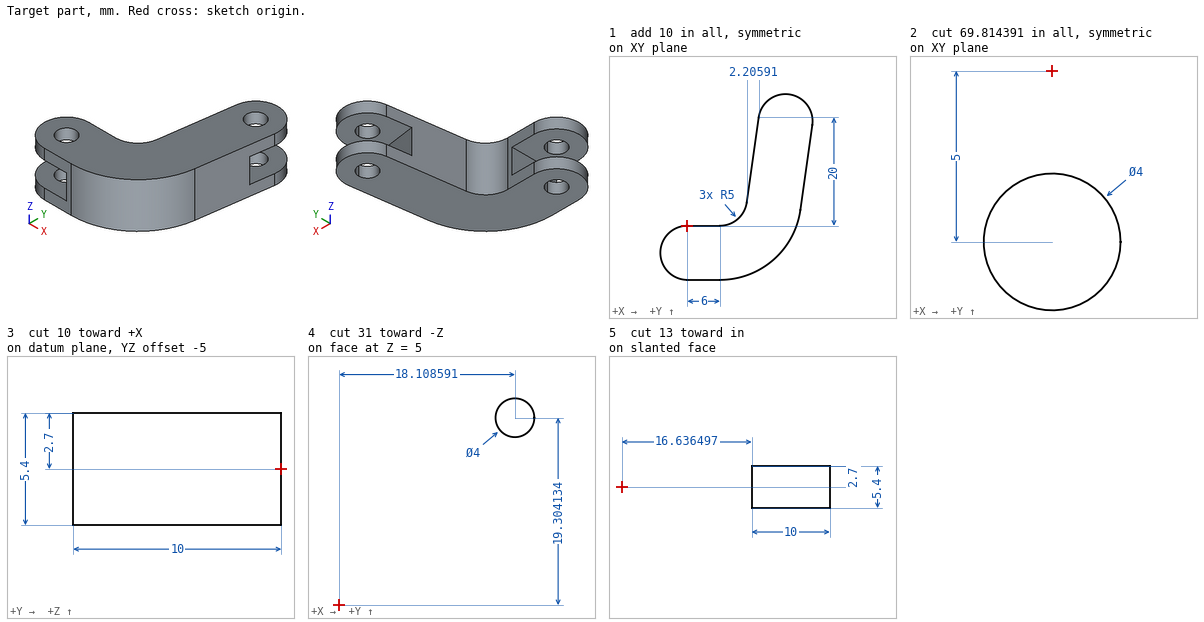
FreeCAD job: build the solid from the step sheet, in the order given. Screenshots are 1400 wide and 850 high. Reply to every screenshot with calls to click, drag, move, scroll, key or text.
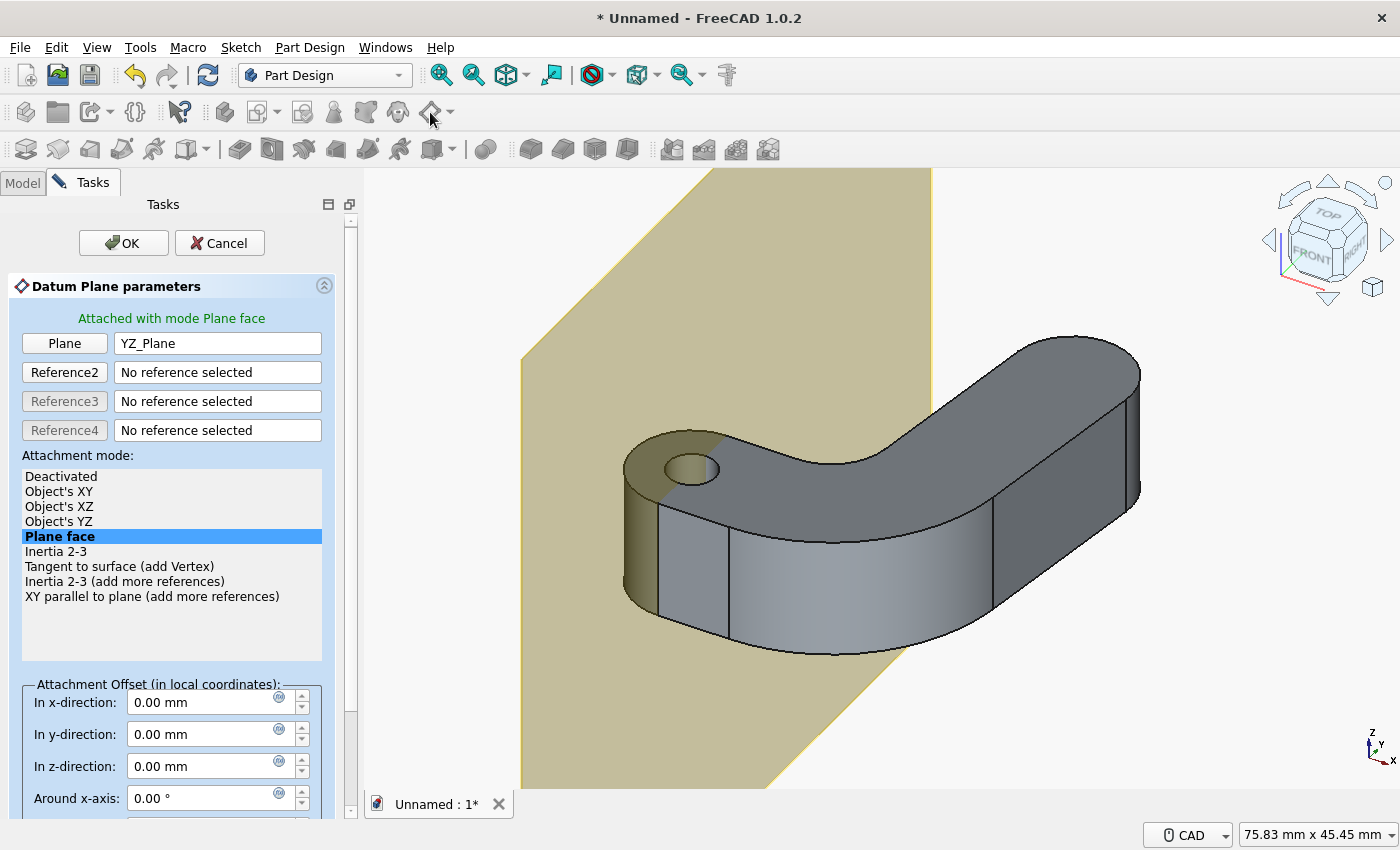
triple_click(210, 766)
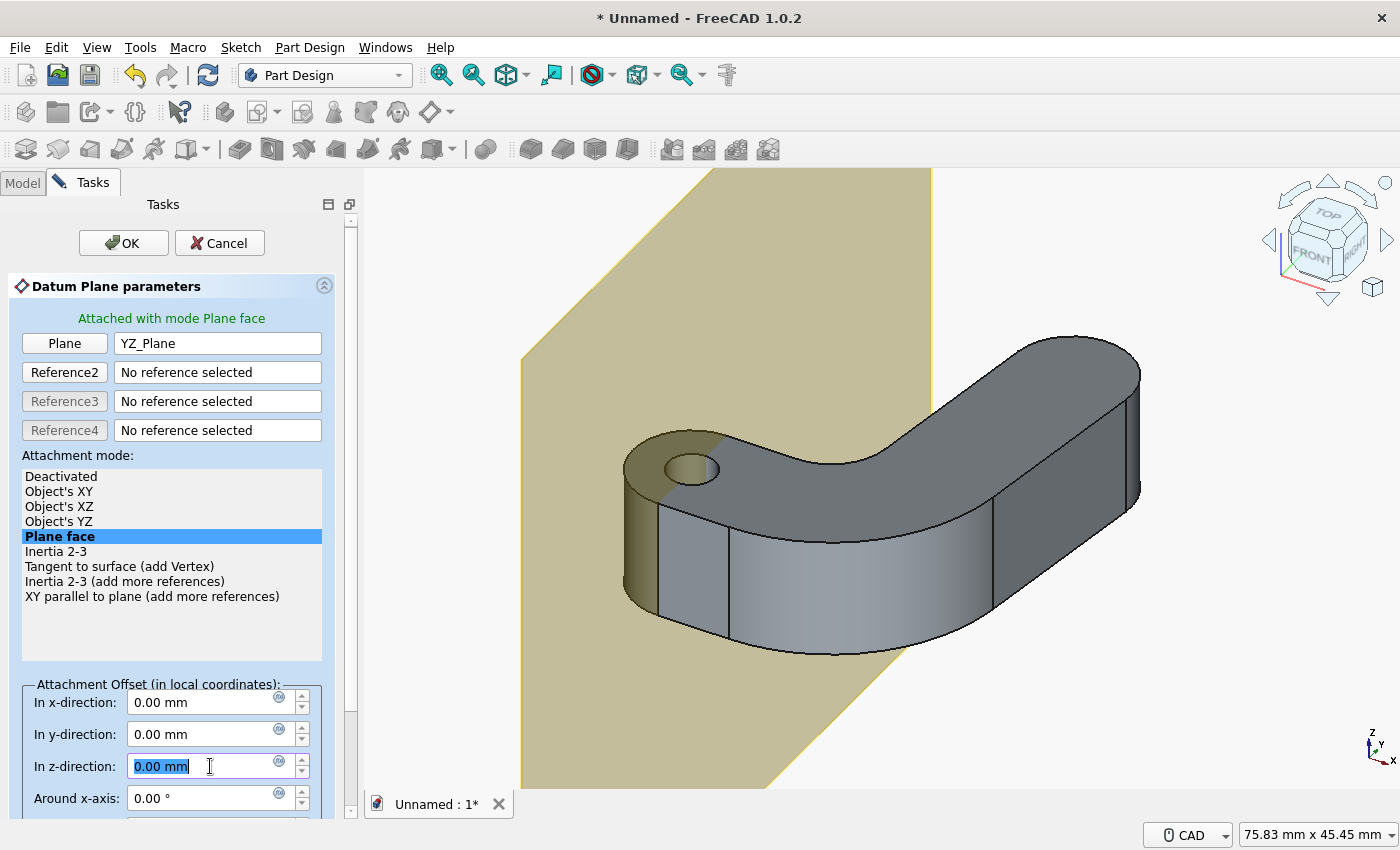
text(-5)
key(Tab)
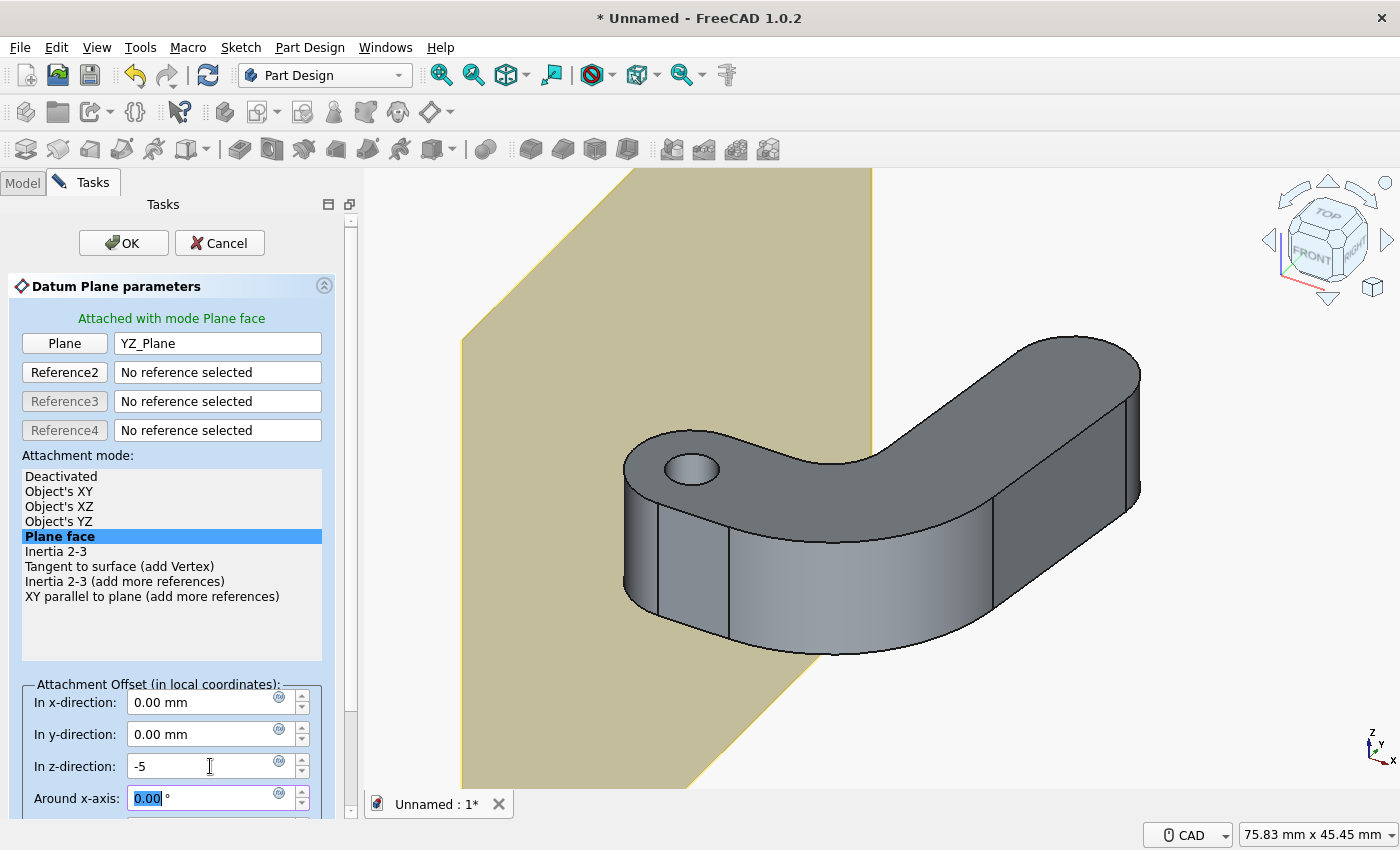
click(124, 243)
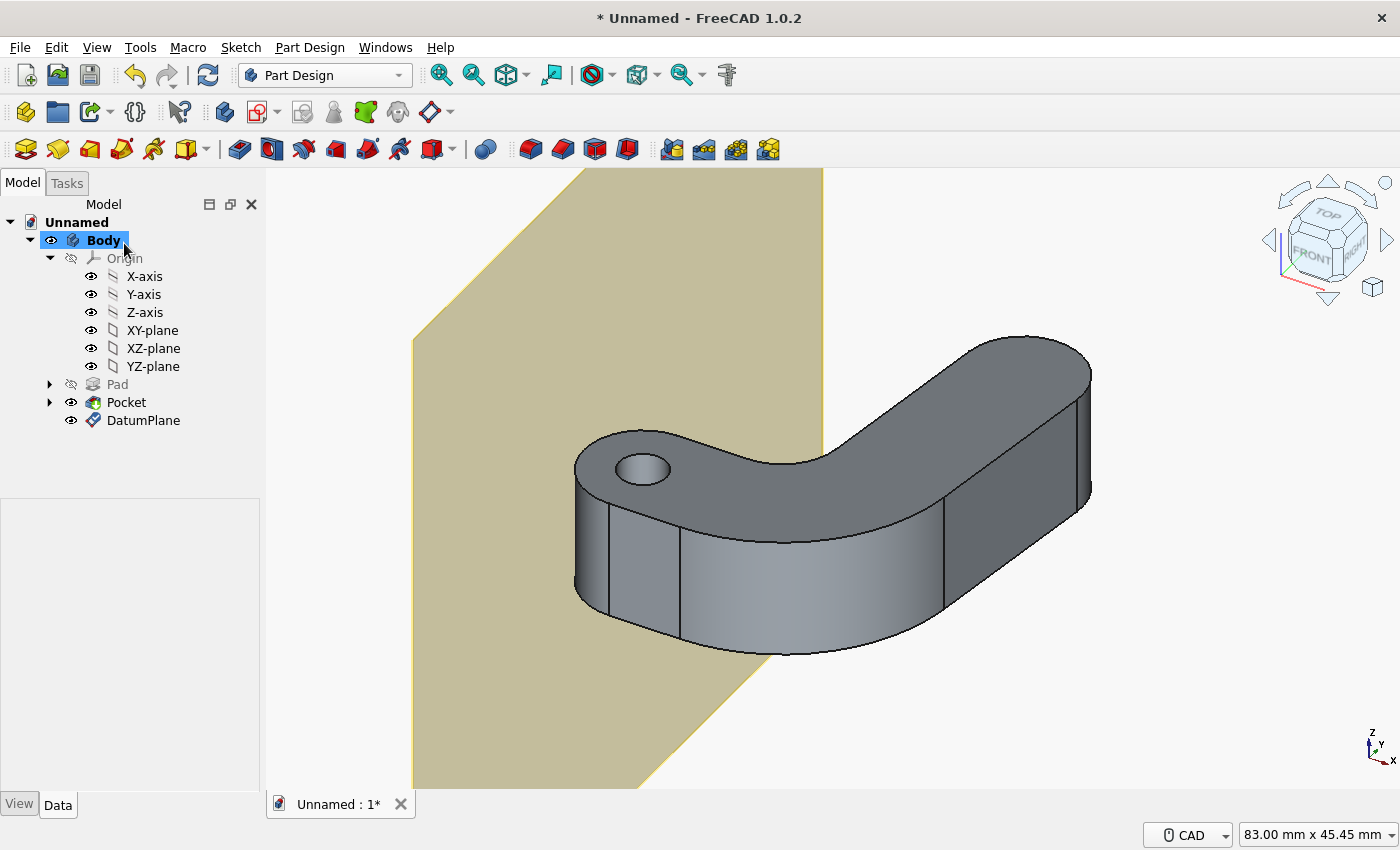
click(116, 420)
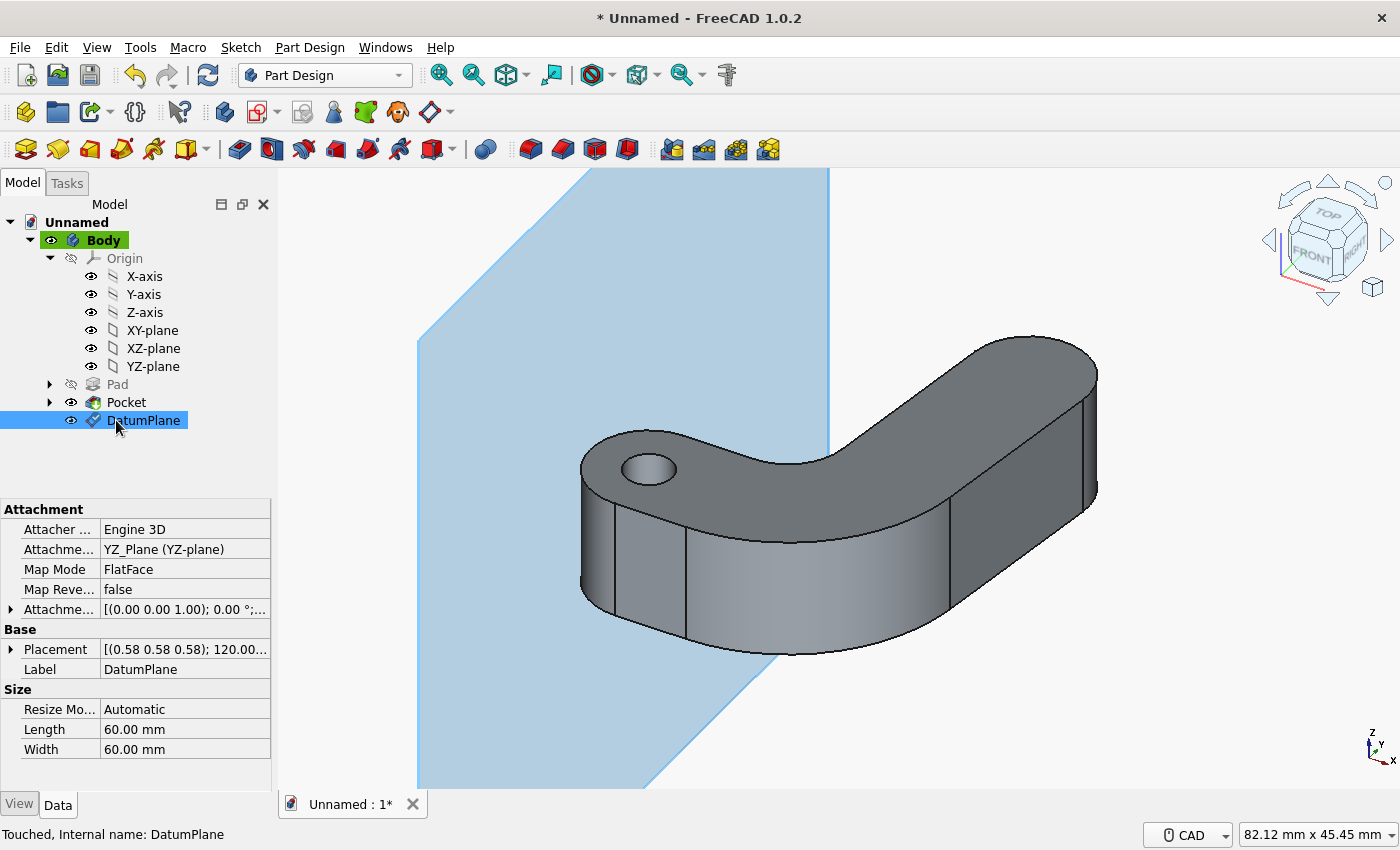
click(258, 112)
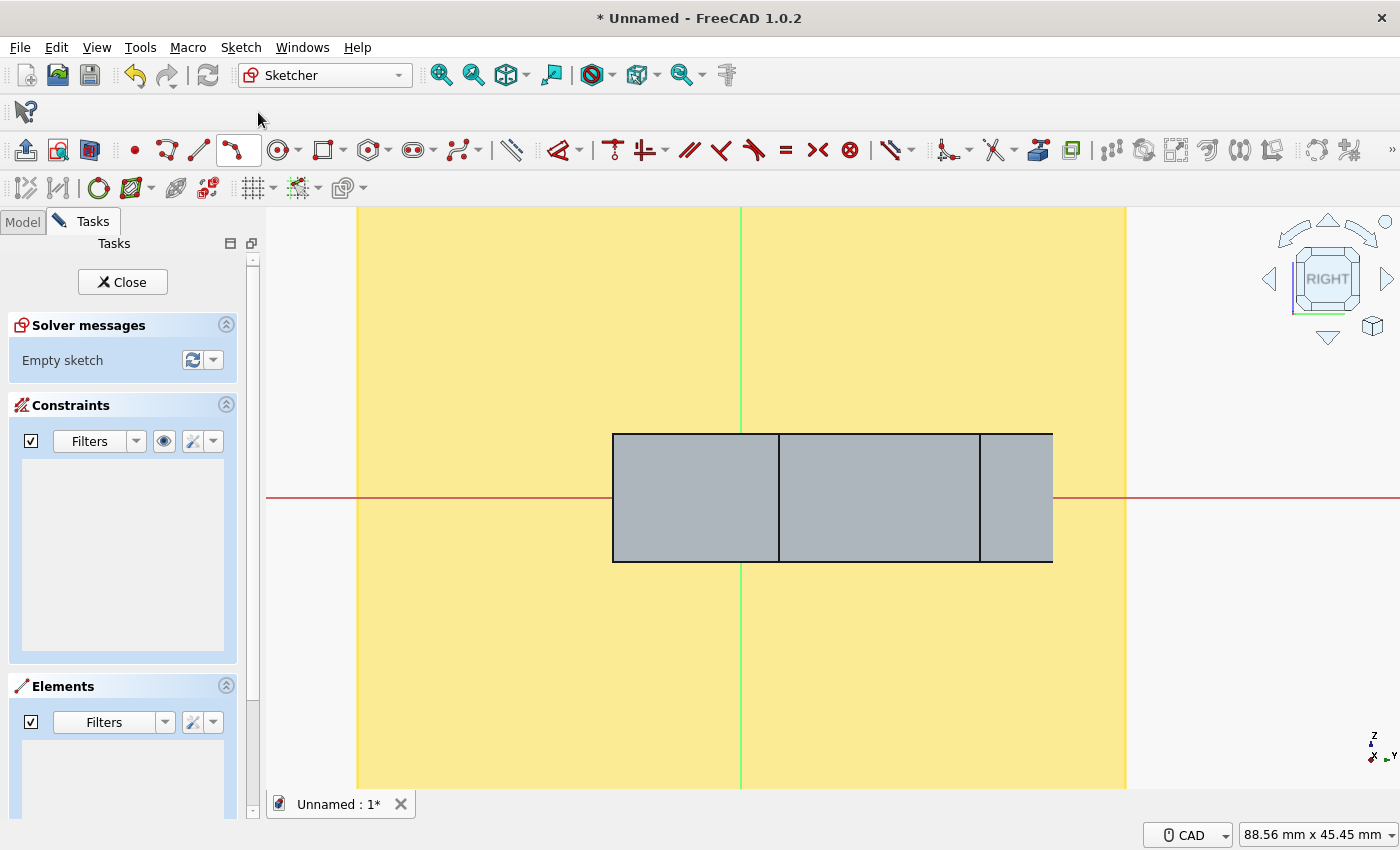
click(90, 150)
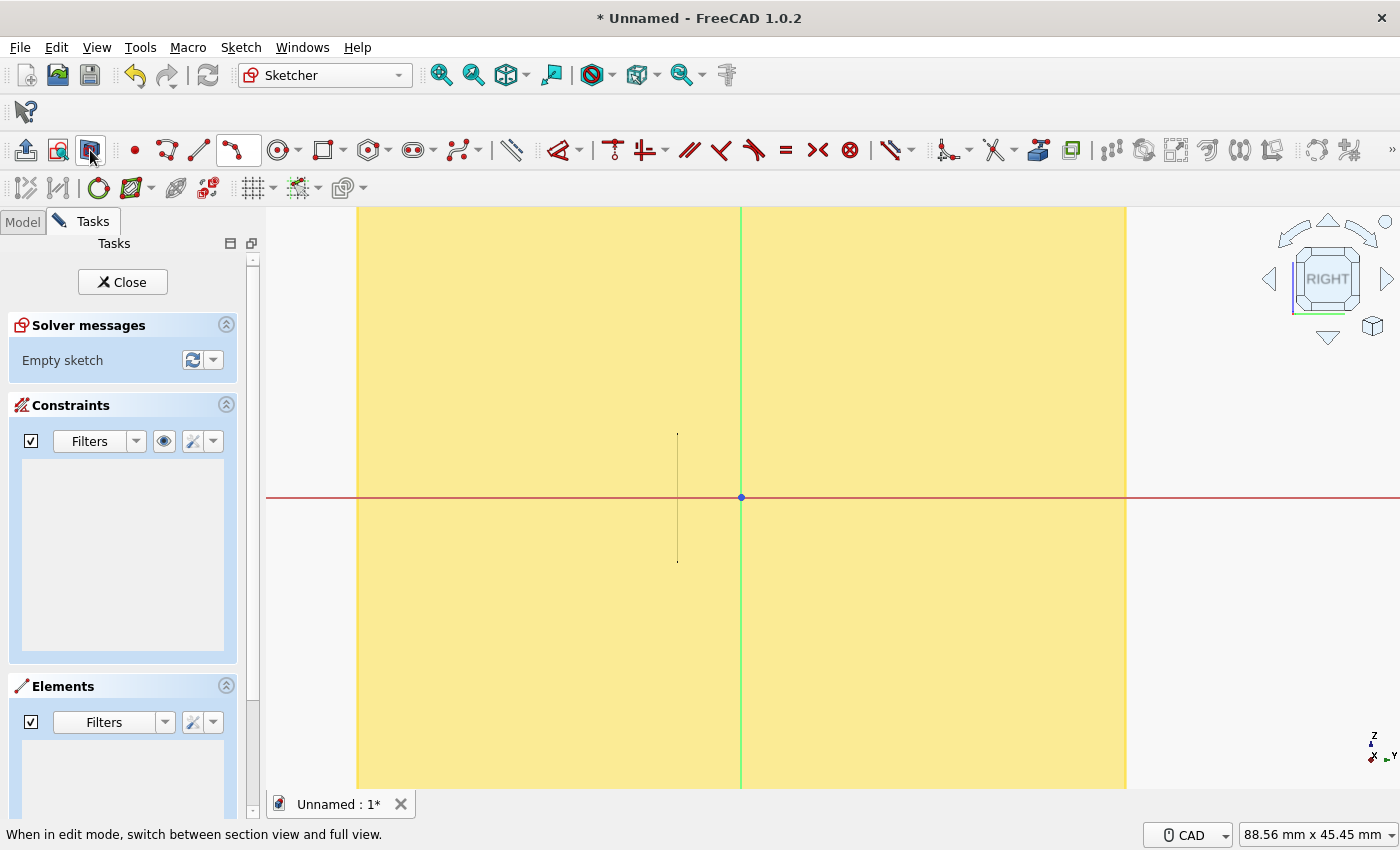
scroll(655, 498, up, 8)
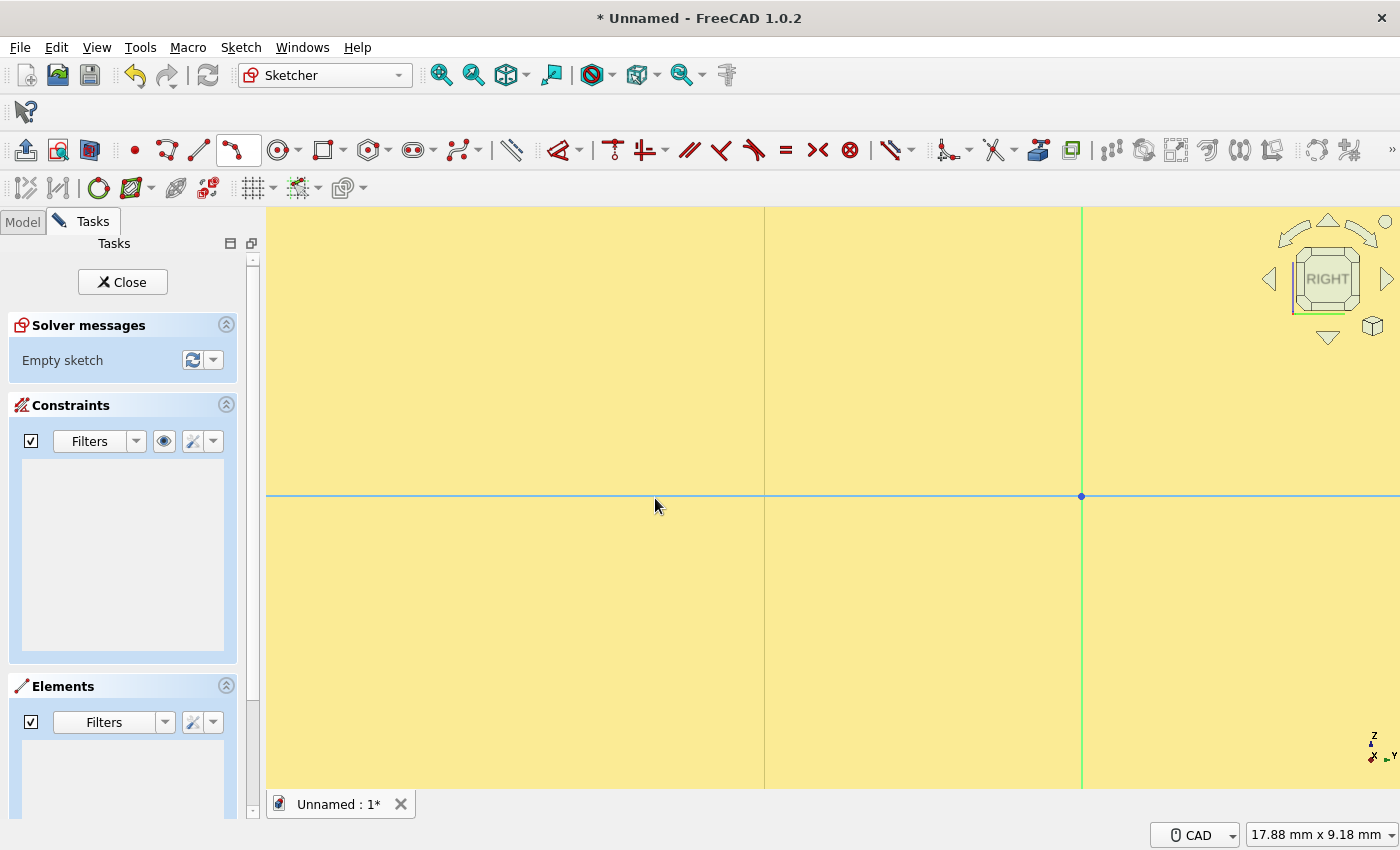
key(g)
key(r)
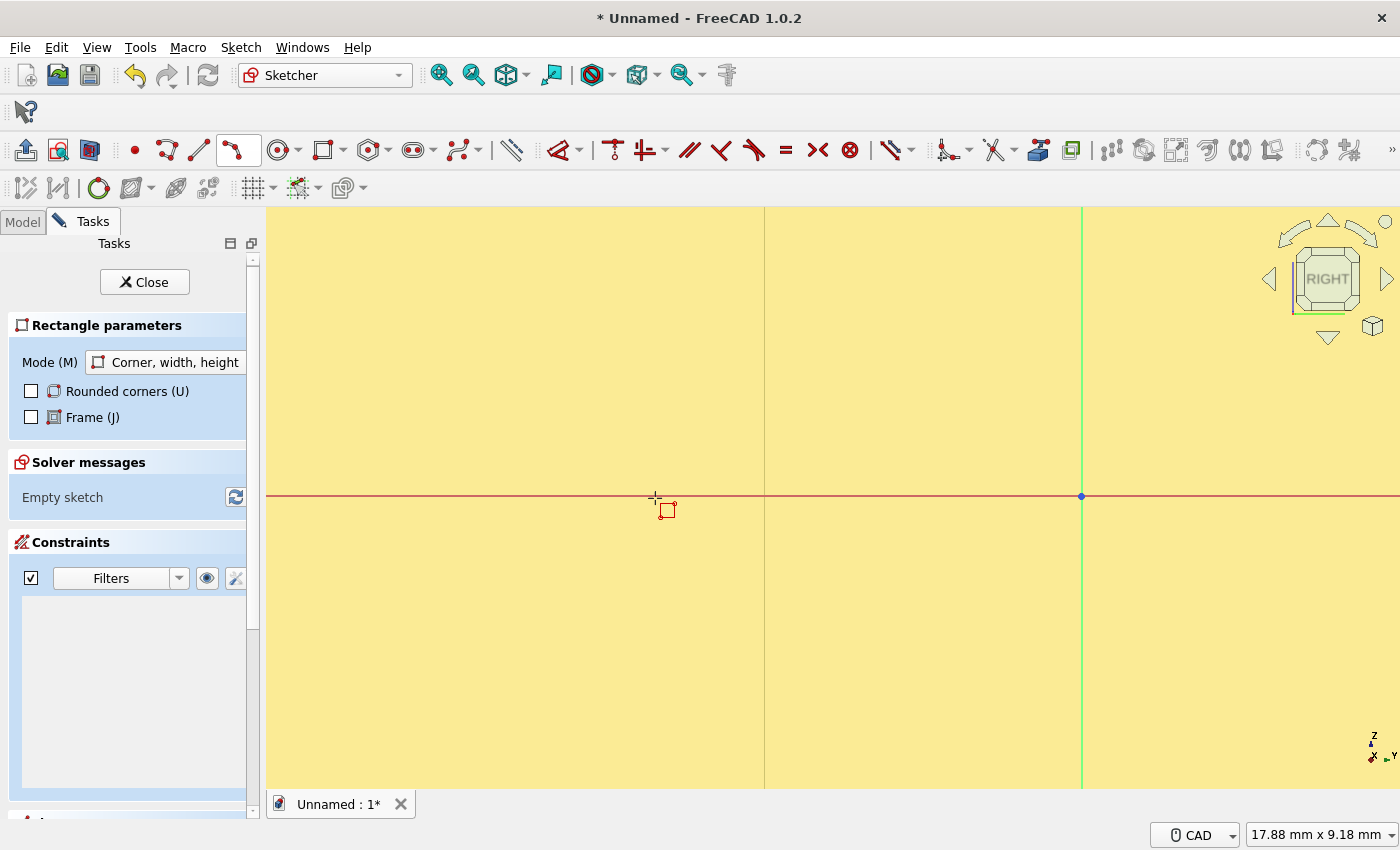
click(448, 325)
click(1082, 667)
key(Escape)